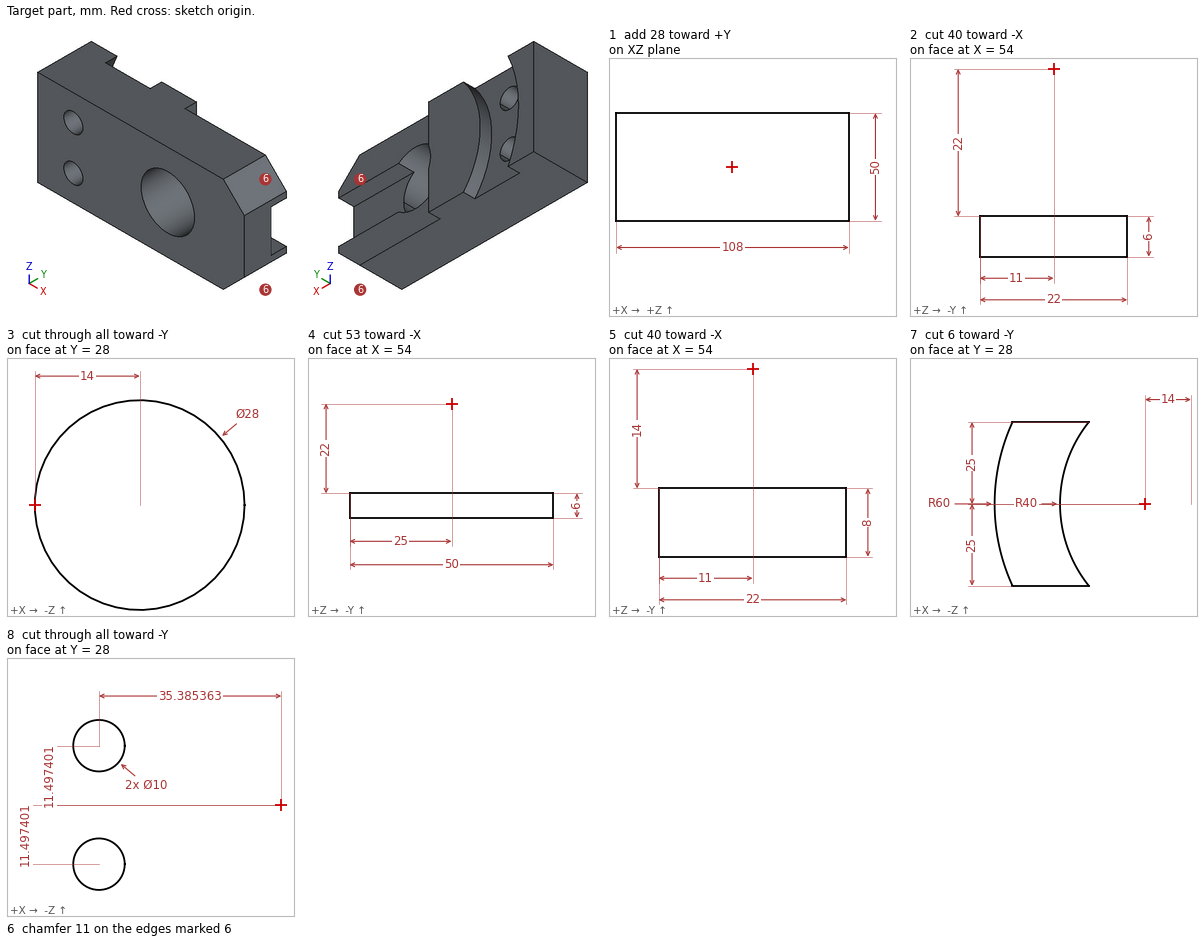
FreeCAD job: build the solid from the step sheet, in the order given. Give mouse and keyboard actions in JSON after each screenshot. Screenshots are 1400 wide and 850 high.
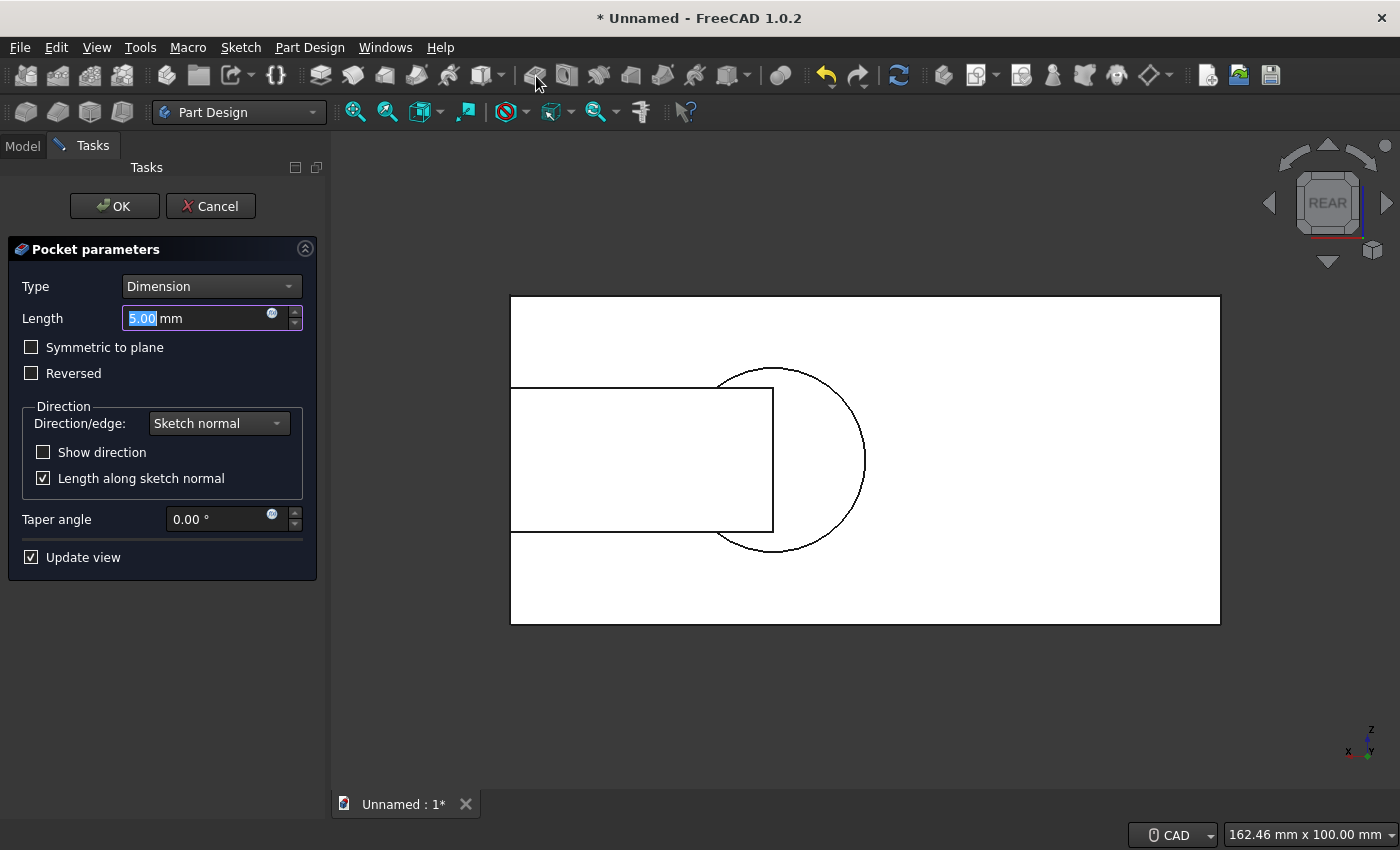
{"action": "left_click", "coordinate": [212, 286]}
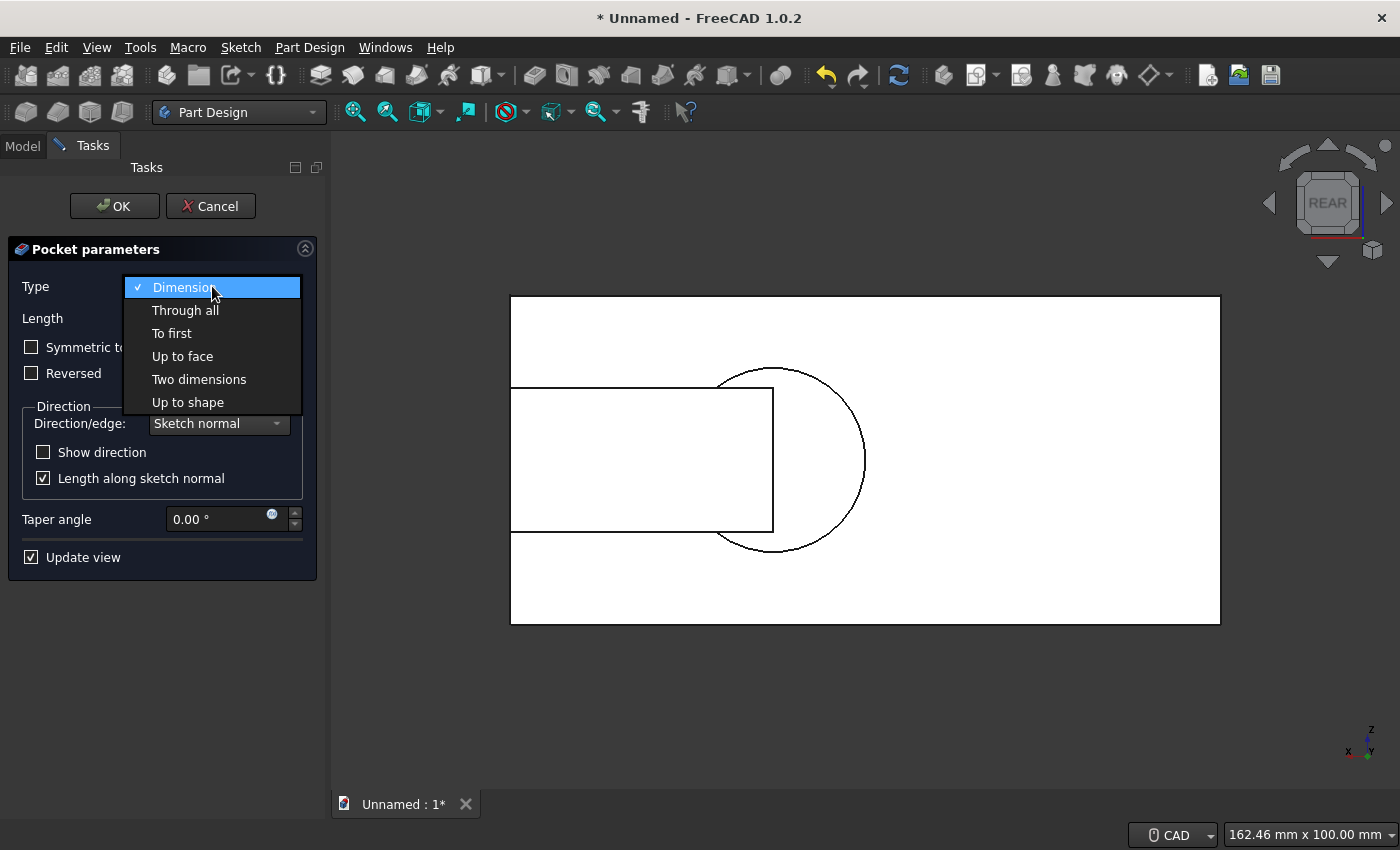
{"action": "left_click", "coordinate": [212, 310]}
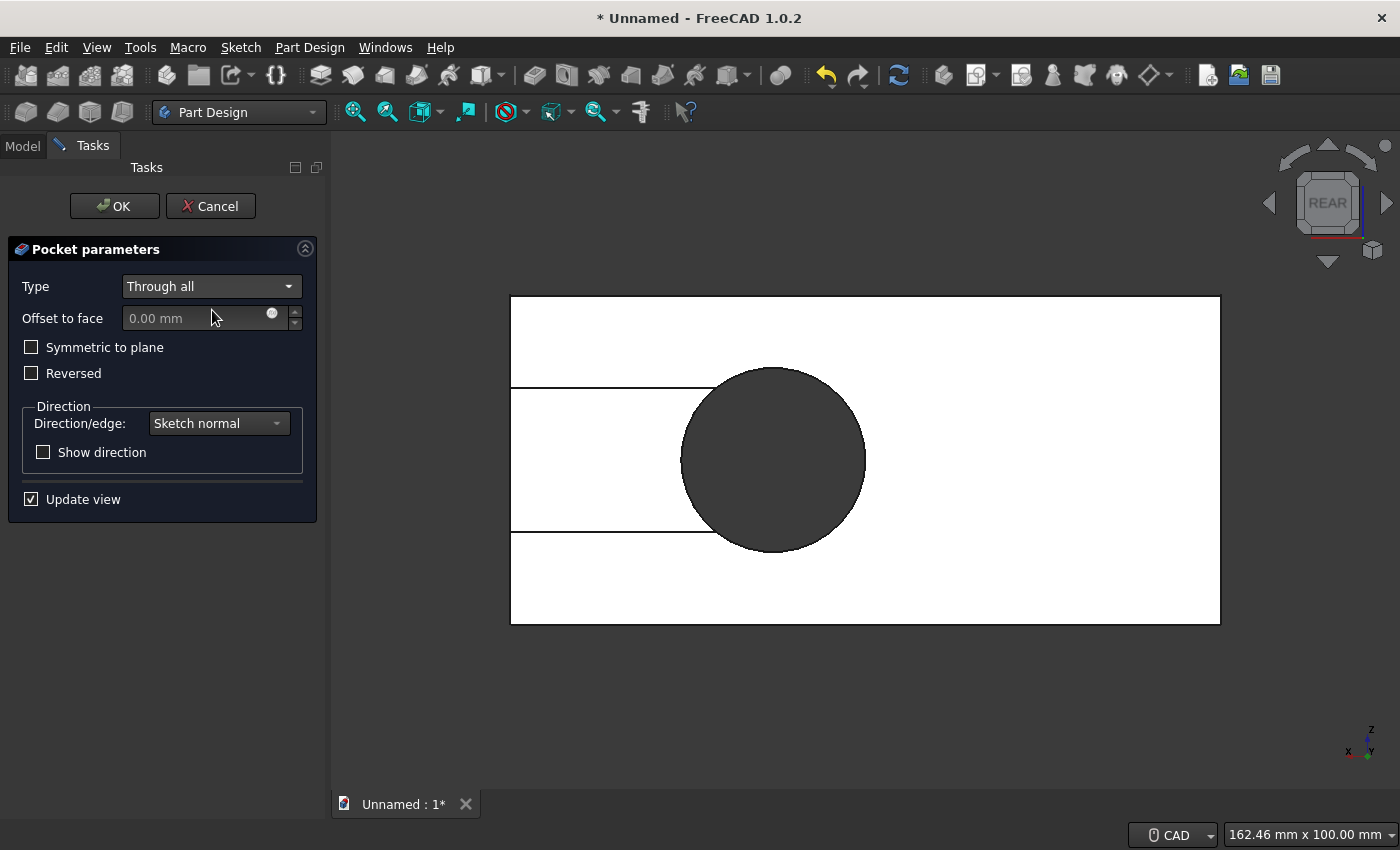
{"action": "left_click", "coordinate": [115, 206]}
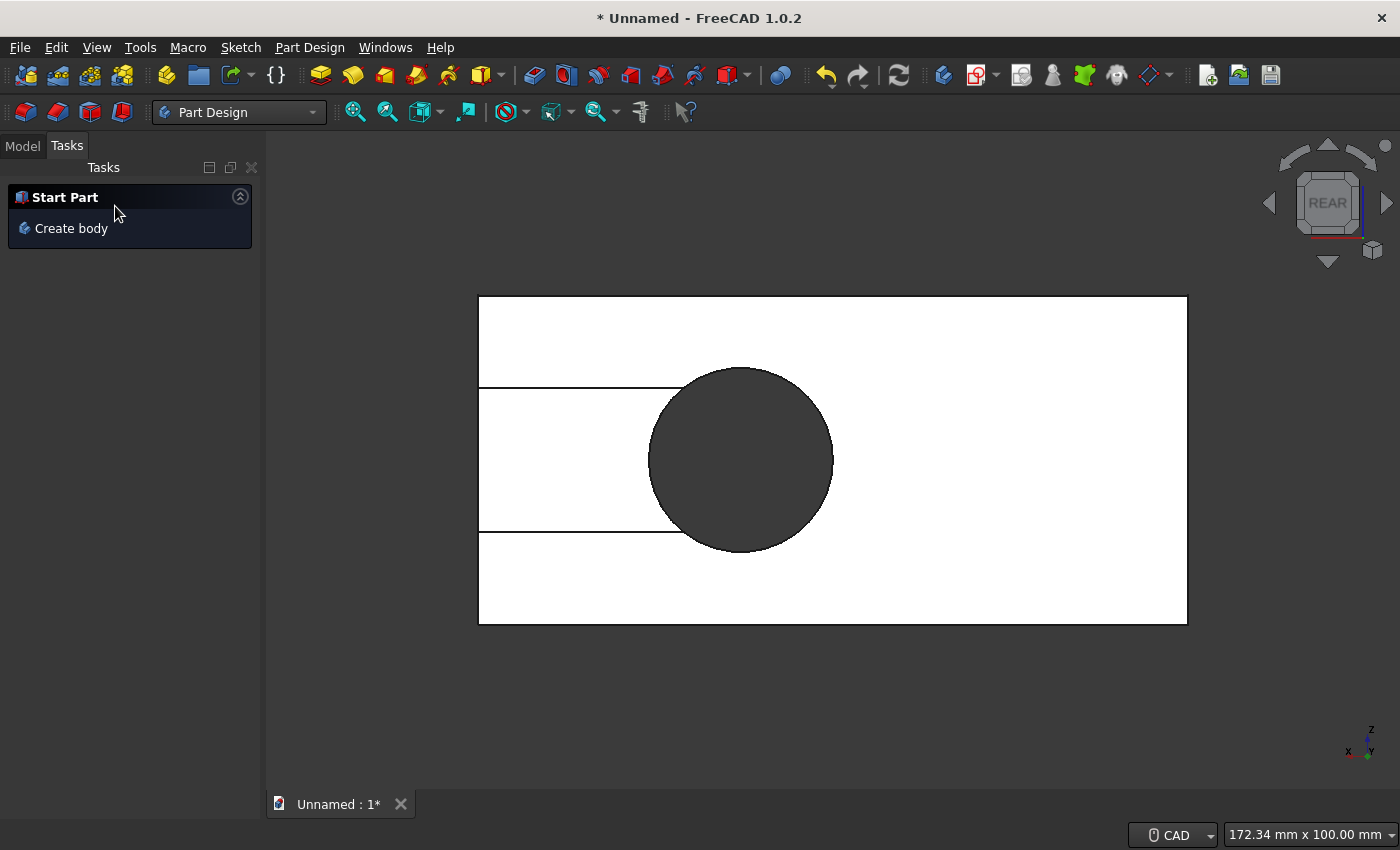
{"action": "key", "text": "0"}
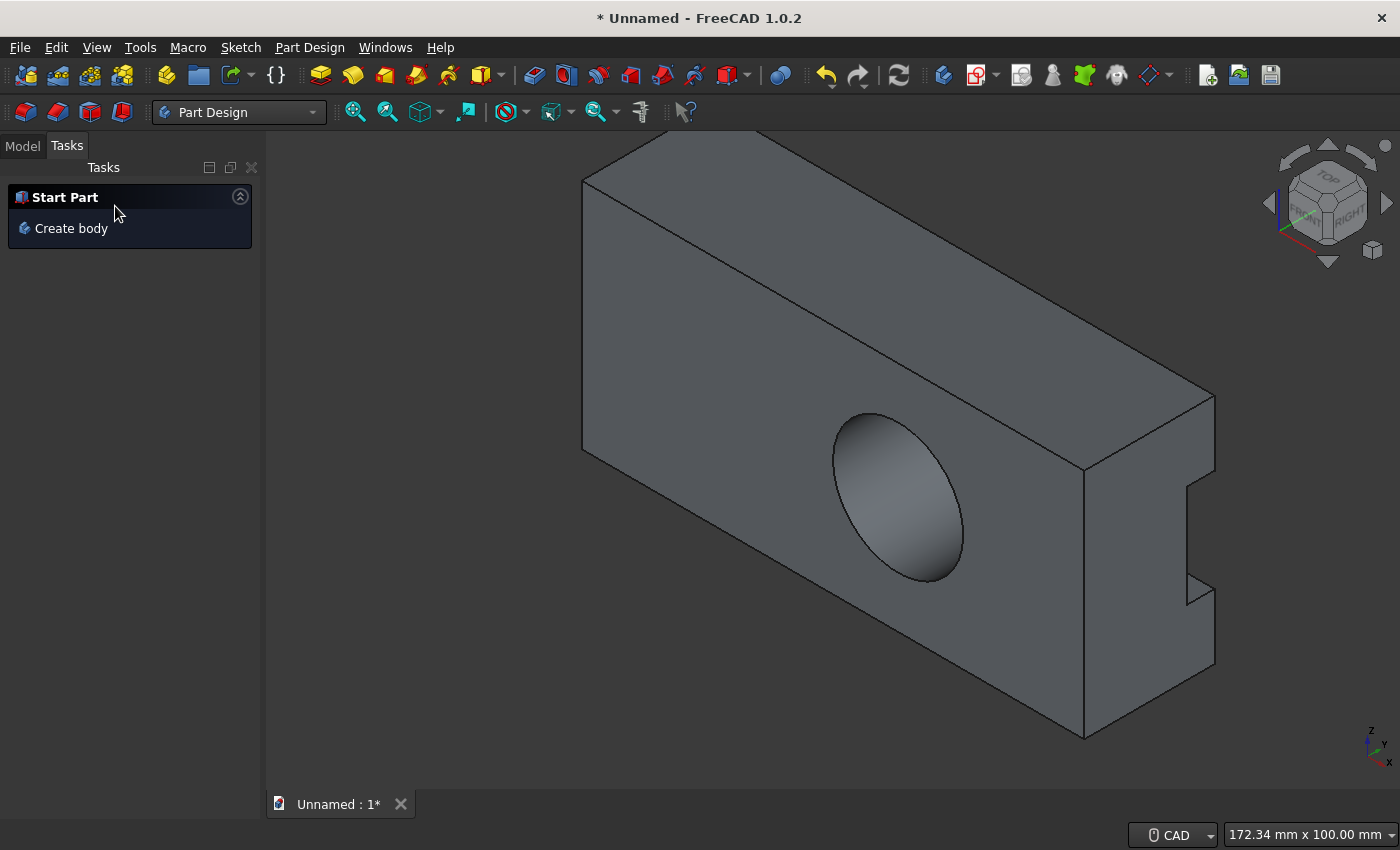
{"action": "key", "text": "v f"}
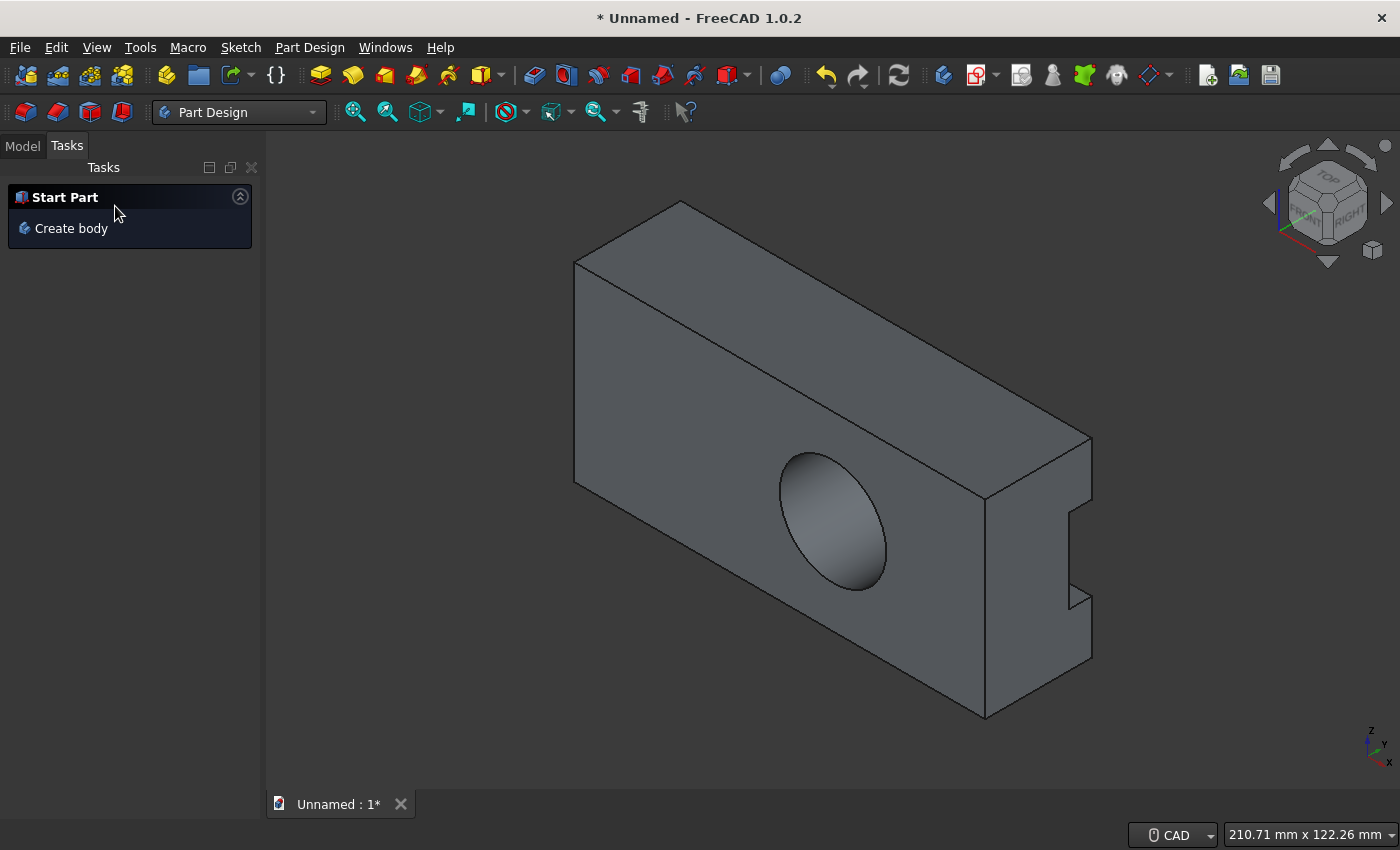
{"action": "left_click", "coordinate": [1023, 649]}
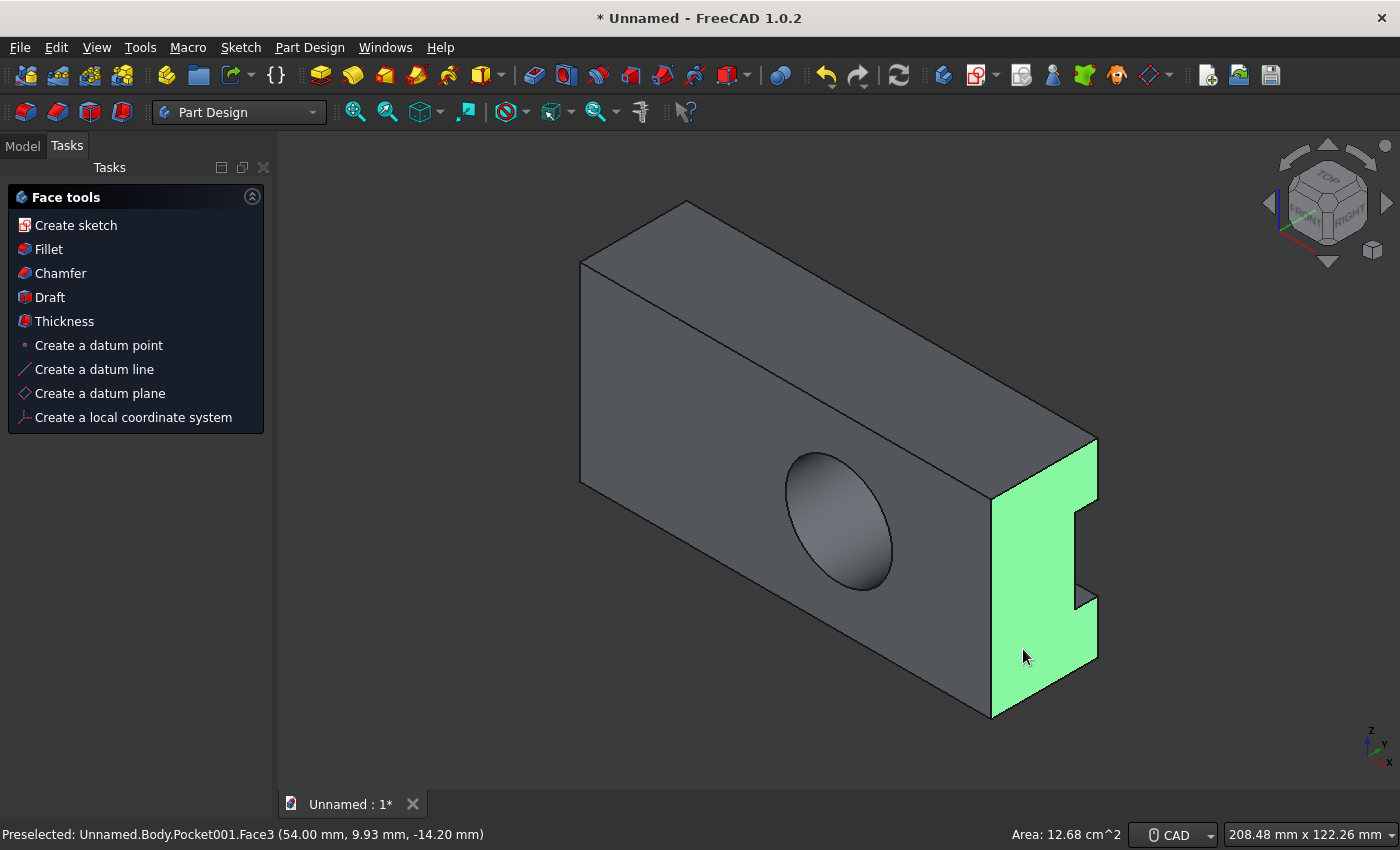
{"action": "left_click", "coordinate": [976, 76]}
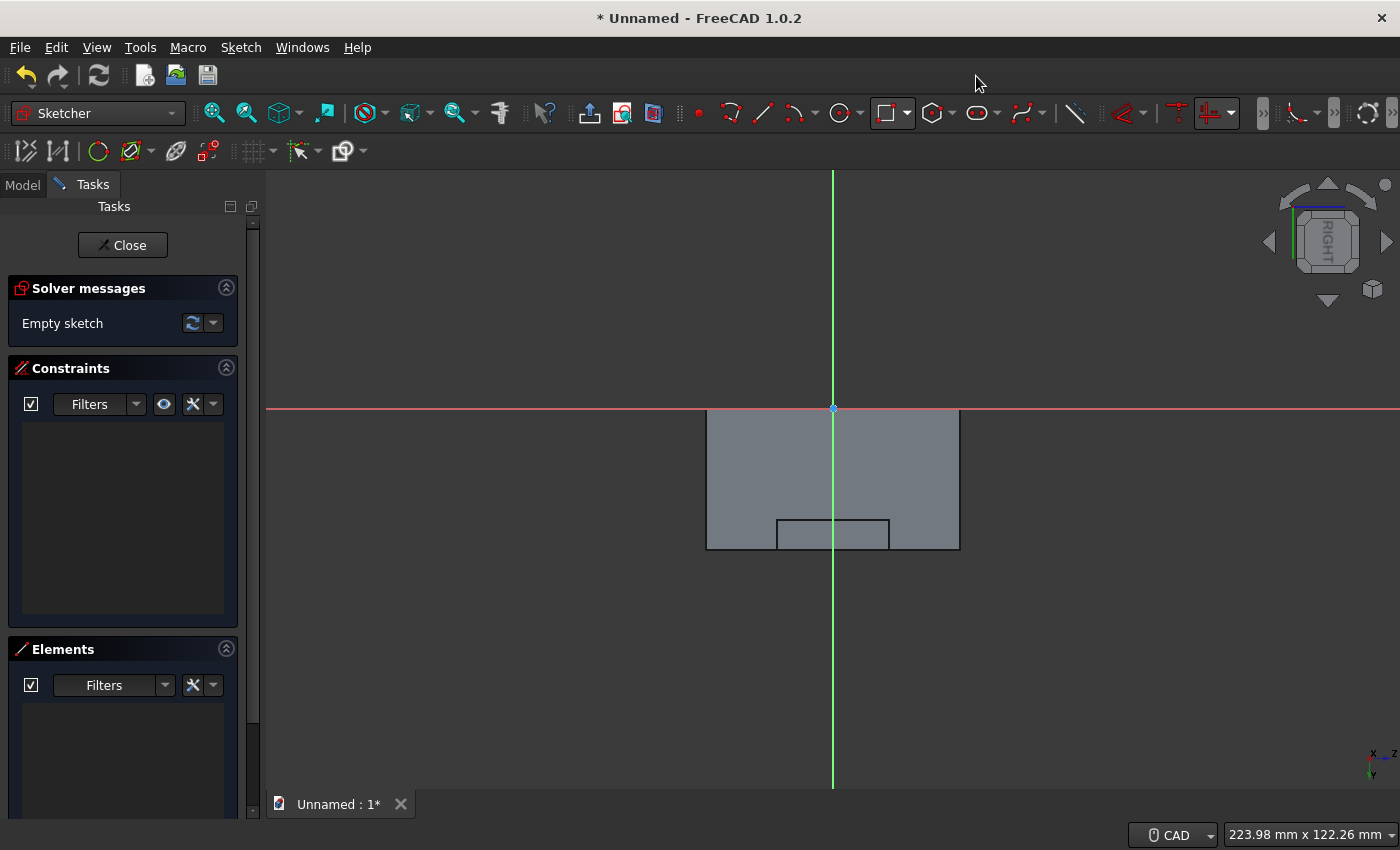
{"action": "scroll", "coordinate": [873, 479], "scroll_direction": "up", "scroll_amount": 5}